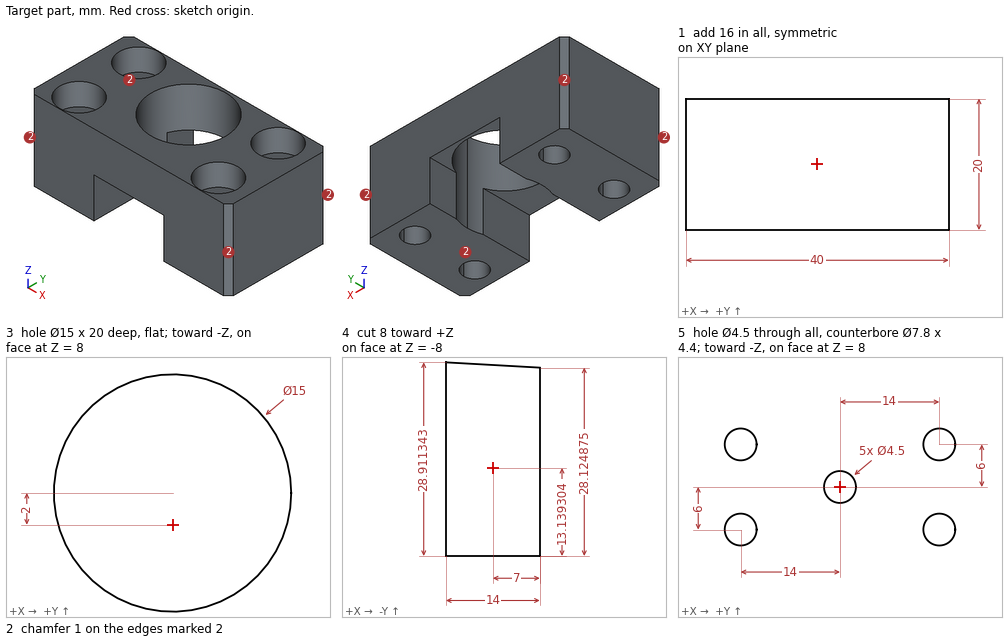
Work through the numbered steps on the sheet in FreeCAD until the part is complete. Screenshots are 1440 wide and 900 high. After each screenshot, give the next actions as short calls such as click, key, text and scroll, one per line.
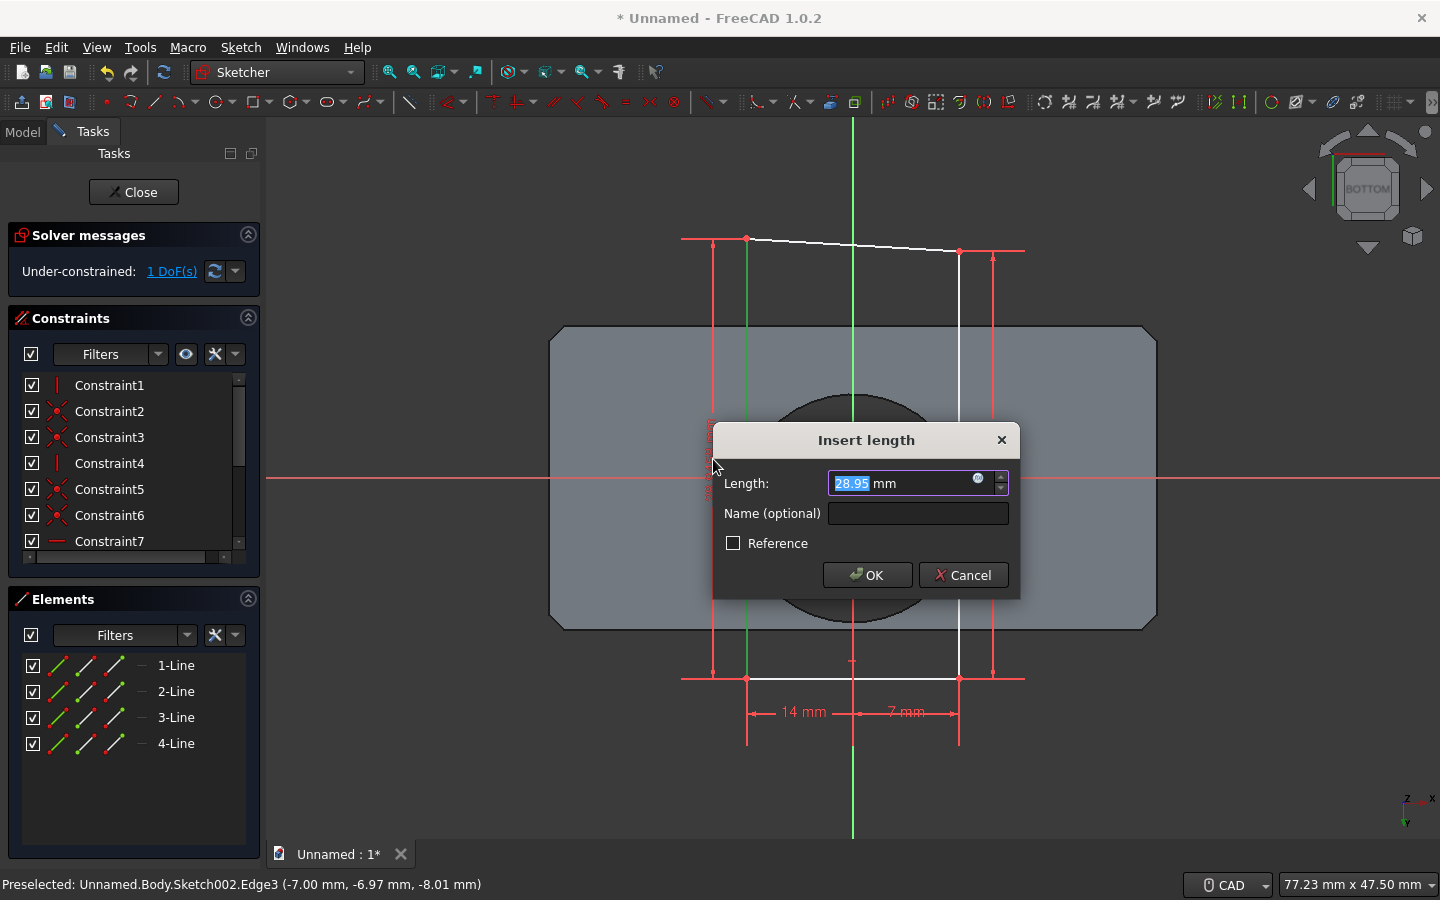
text(28.911343)
key(Return)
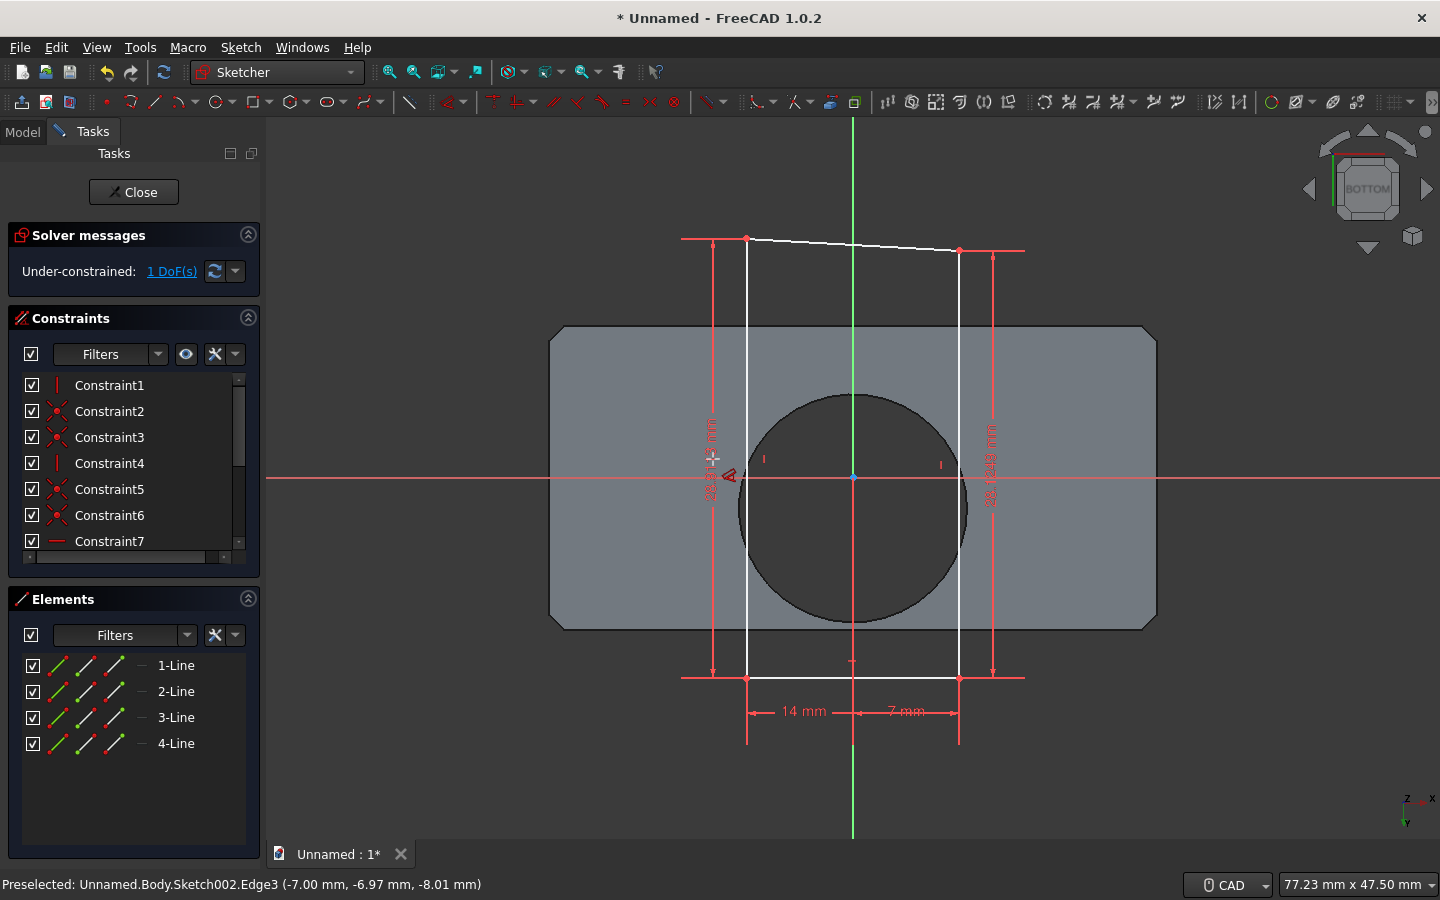
click(959, 678)
click(993, 578)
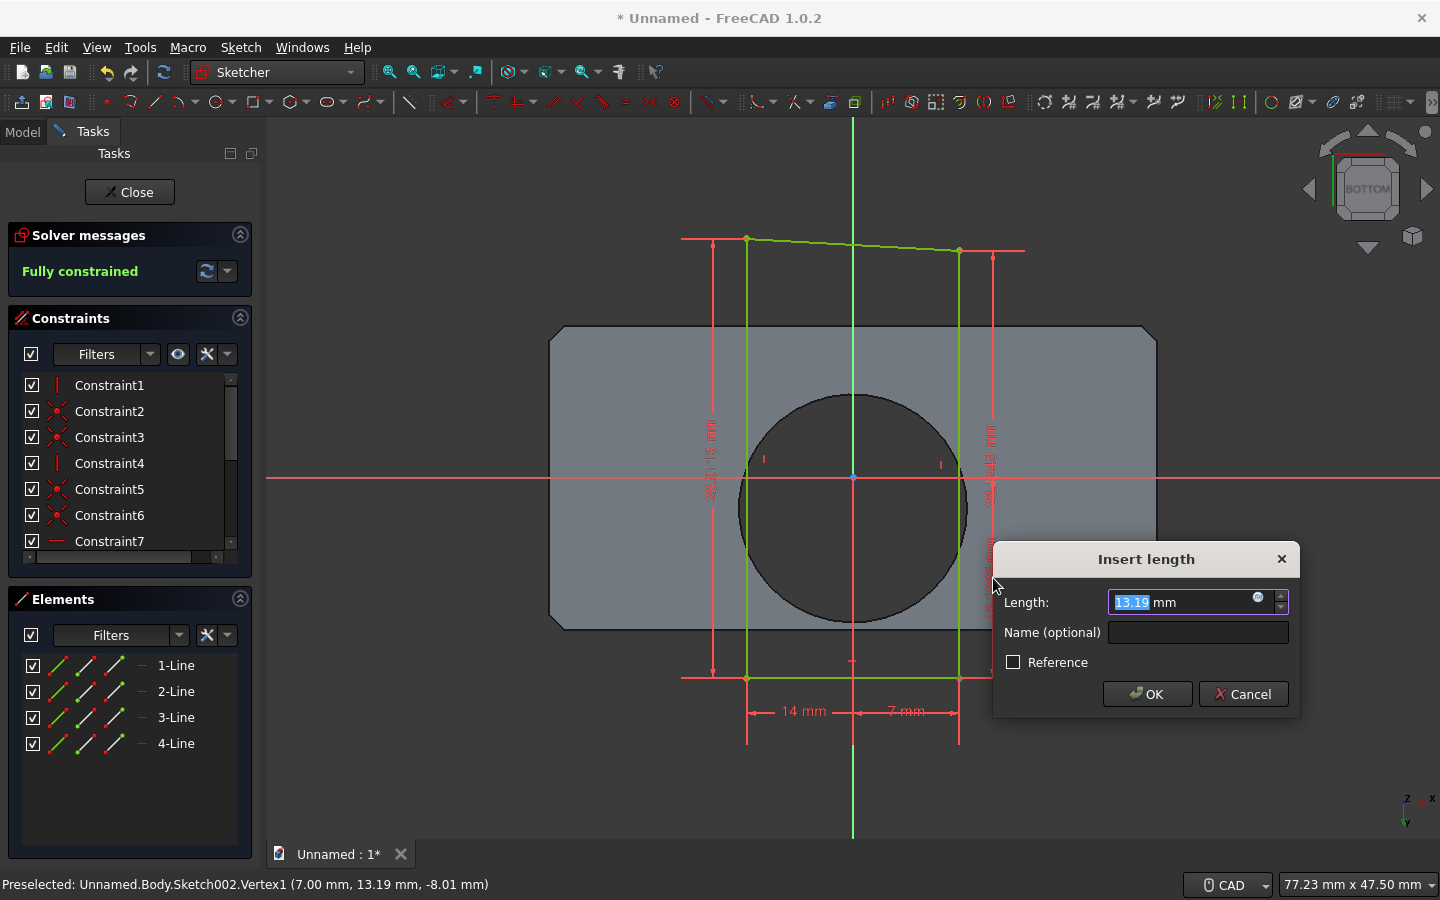
text(13.139304)
key(Return)
key(Escape)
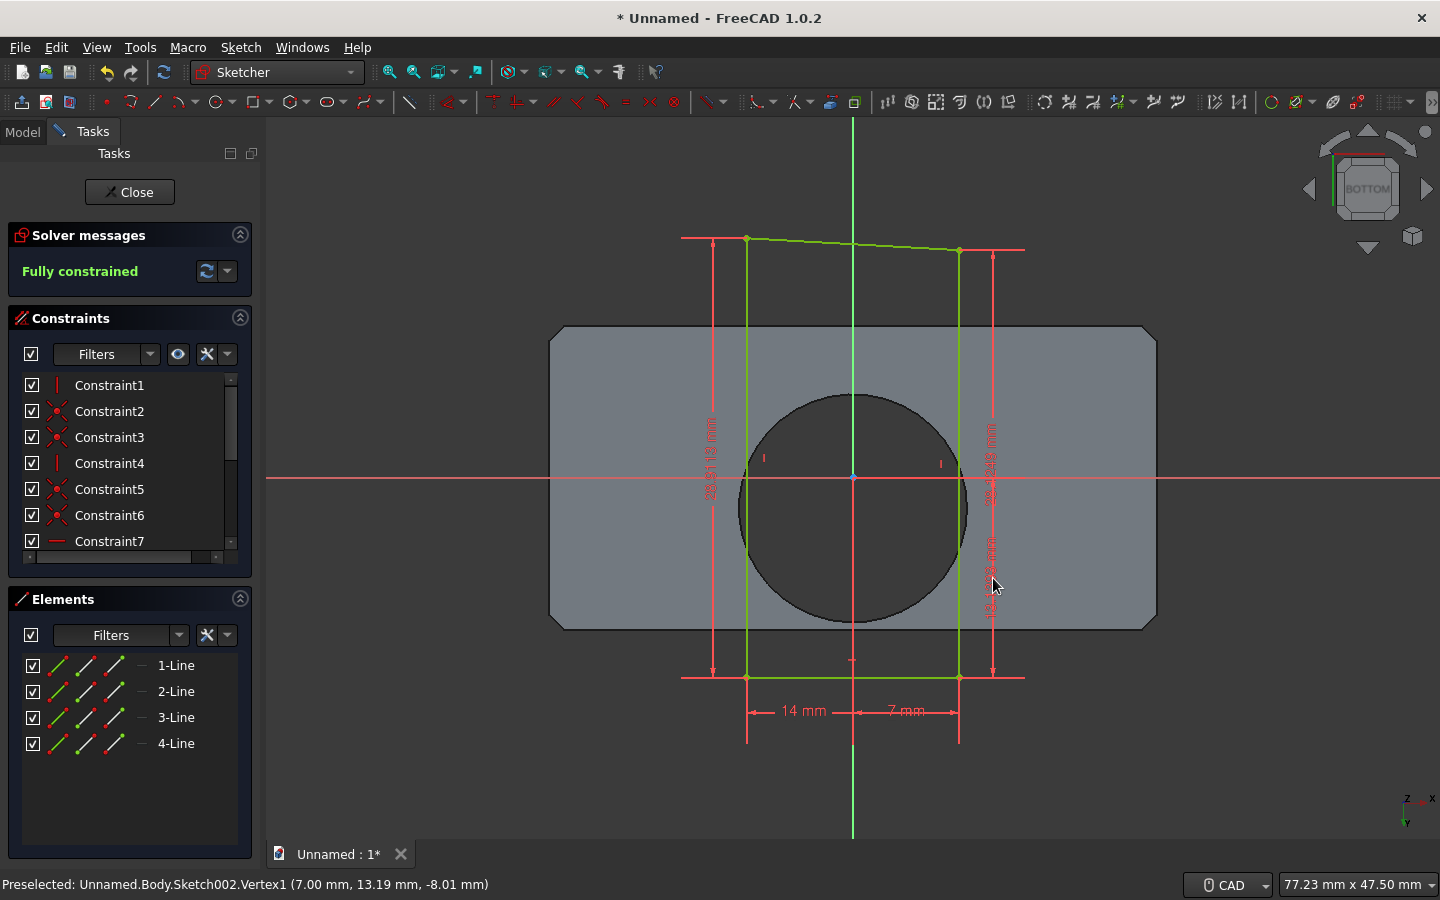
click(130, 192)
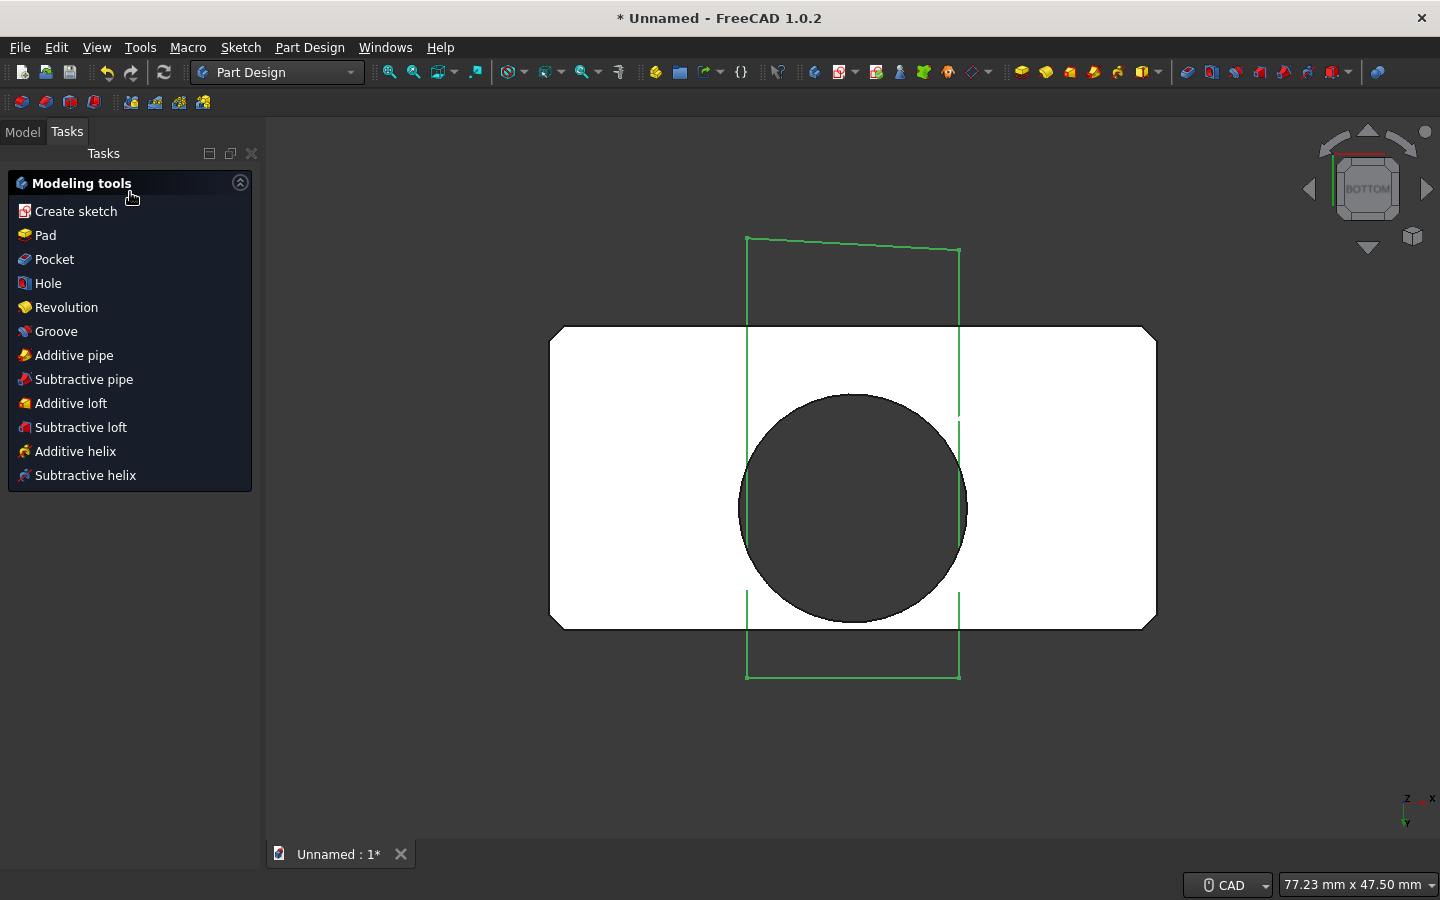
click(1188, 72)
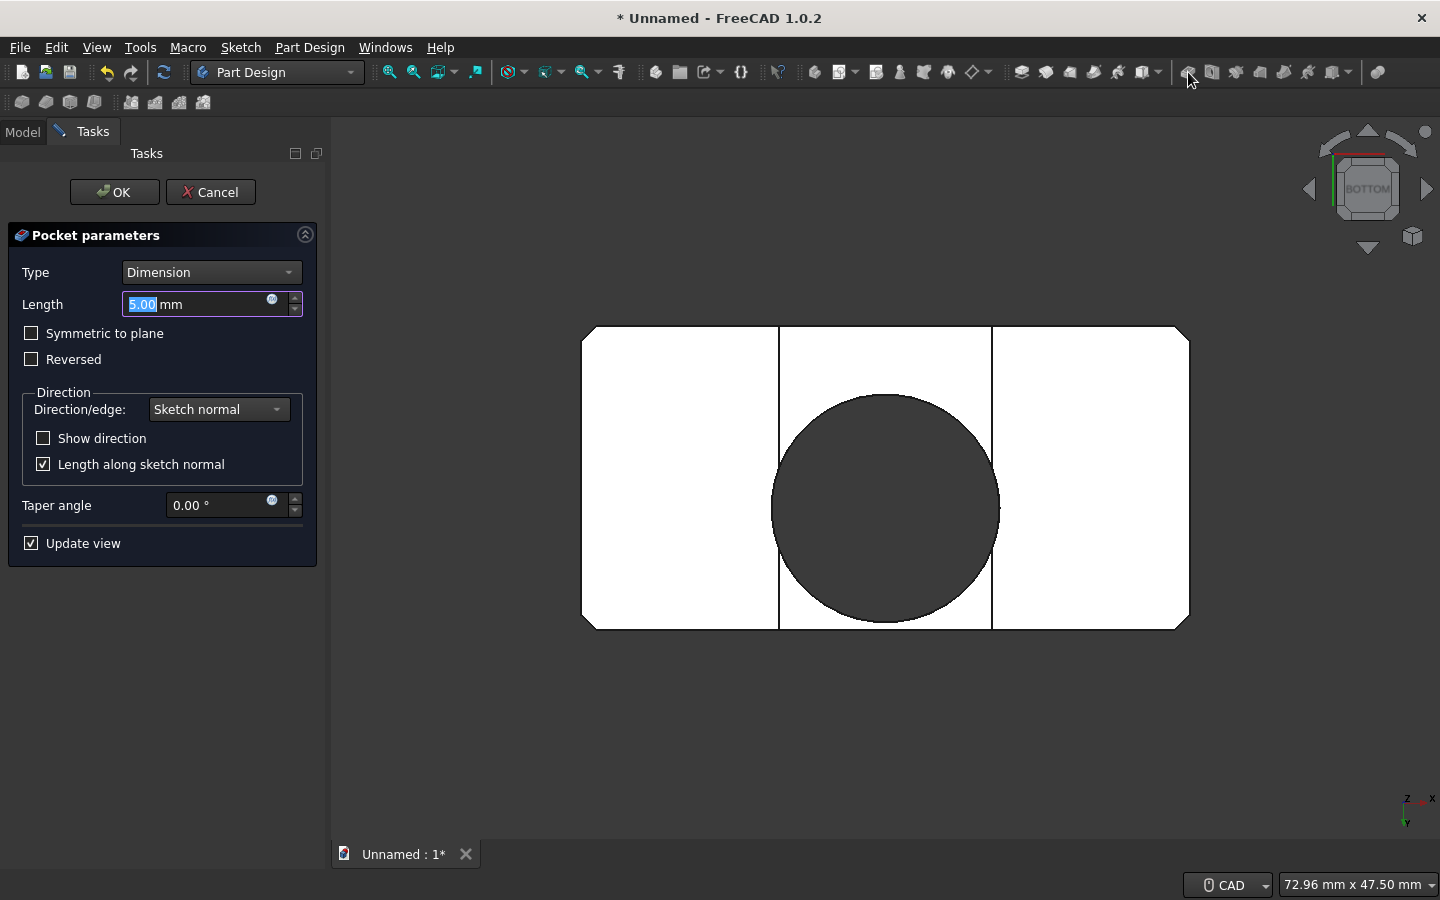
text(8)
key(Tab)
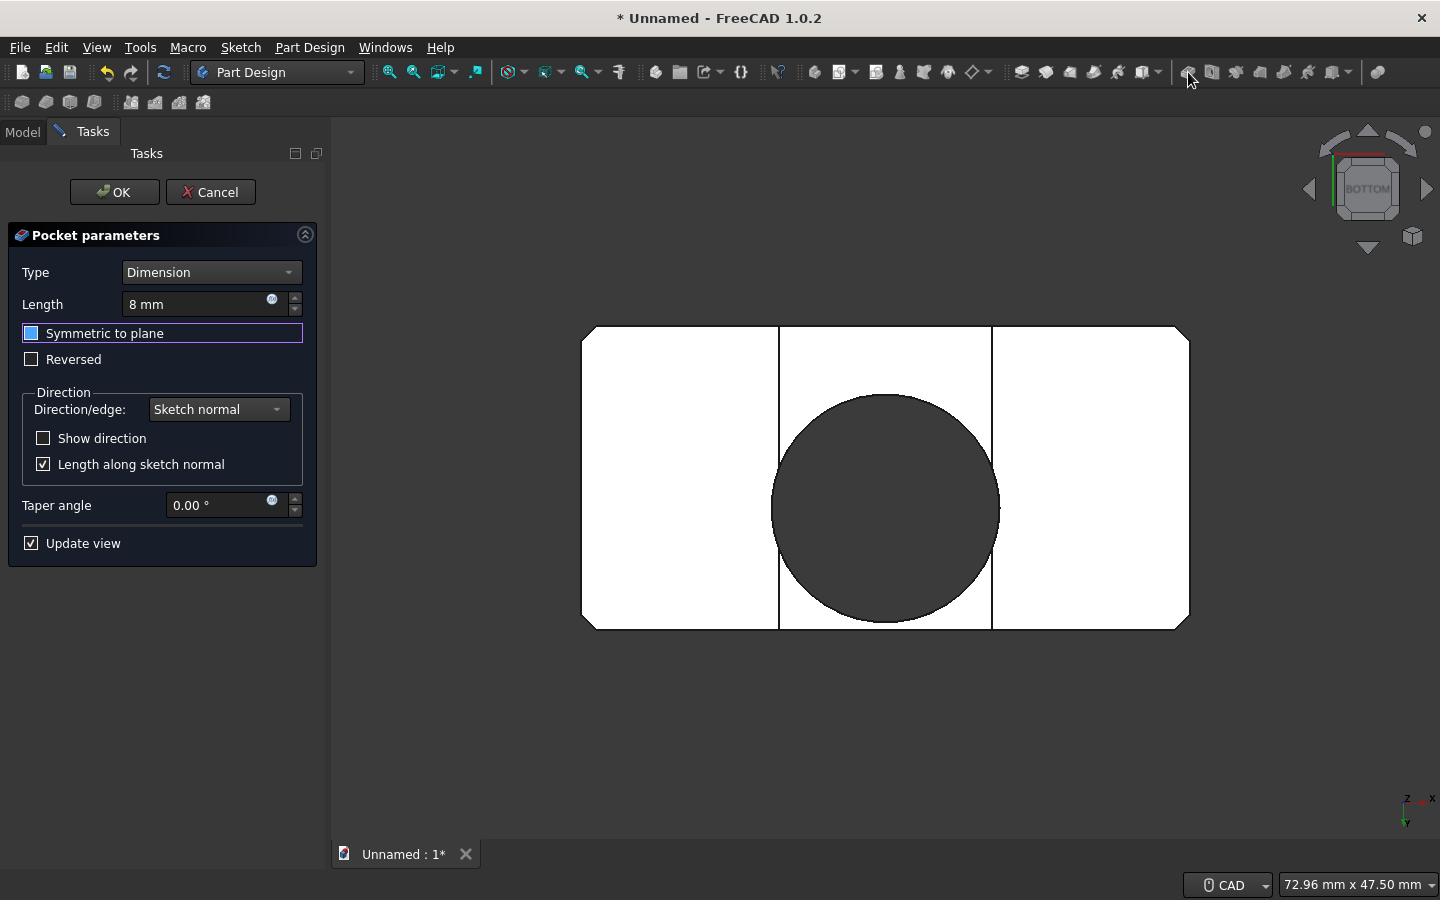
click(115, 192)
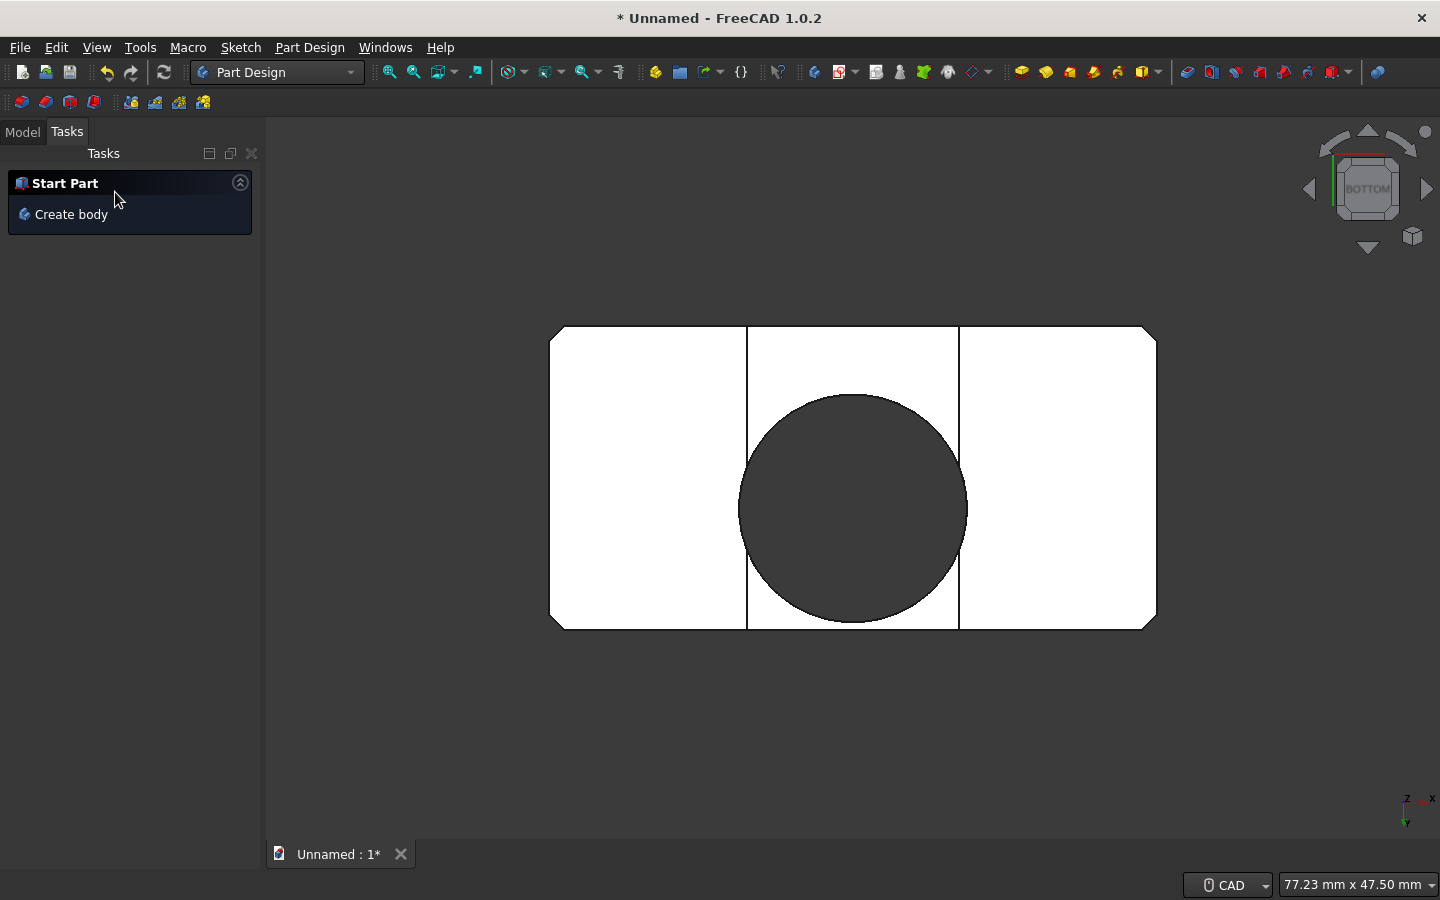
key(0)